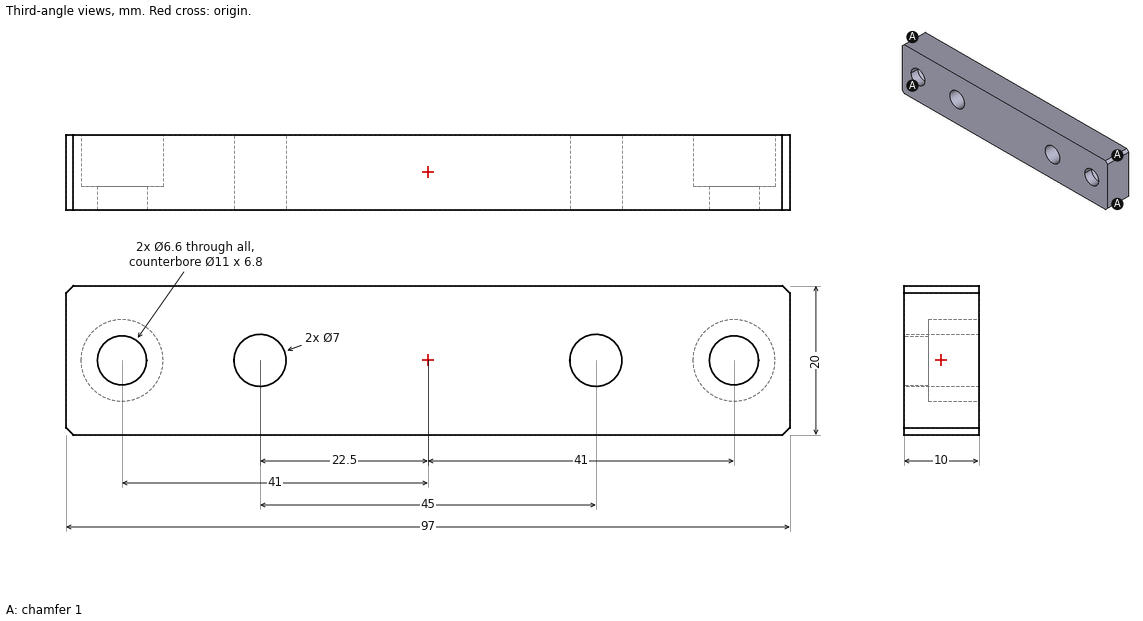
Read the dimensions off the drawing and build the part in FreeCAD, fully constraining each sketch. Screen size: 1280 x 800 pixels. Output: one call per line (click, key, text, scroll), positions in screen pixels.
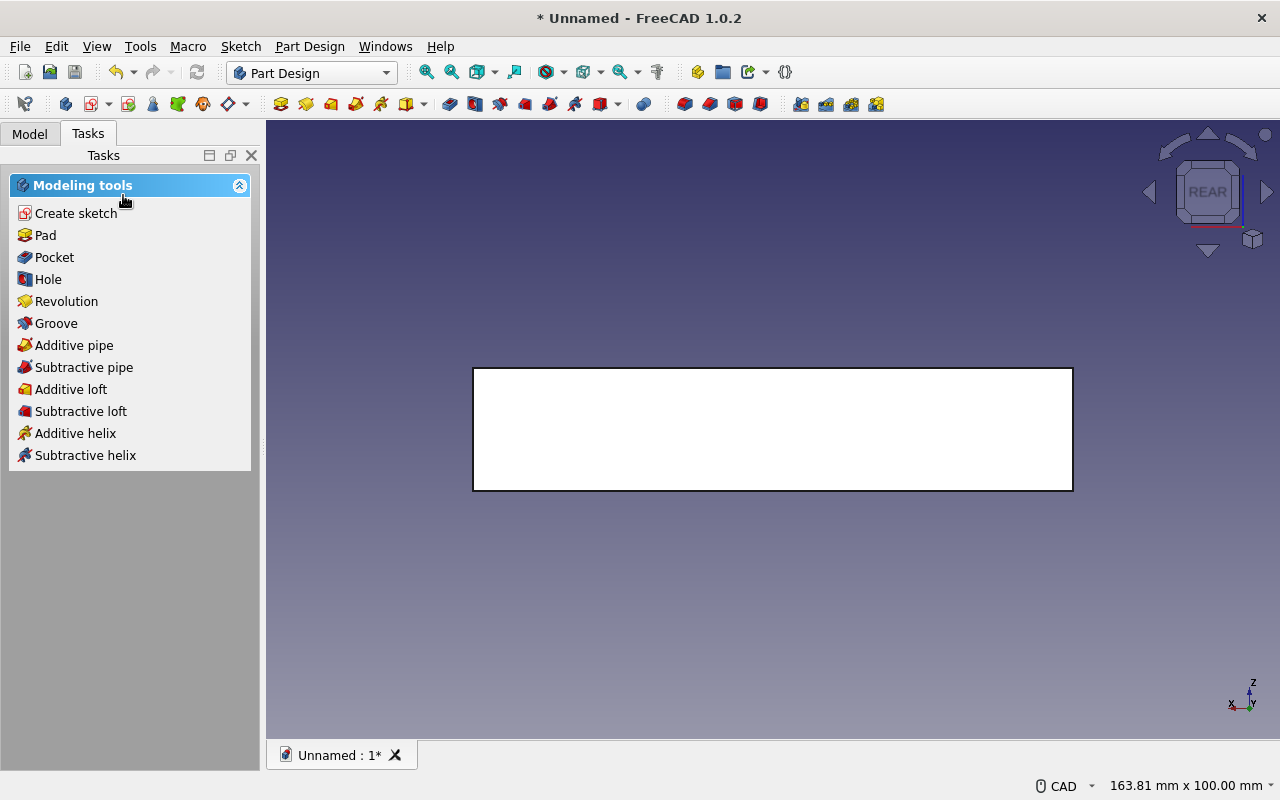
click(450, 104)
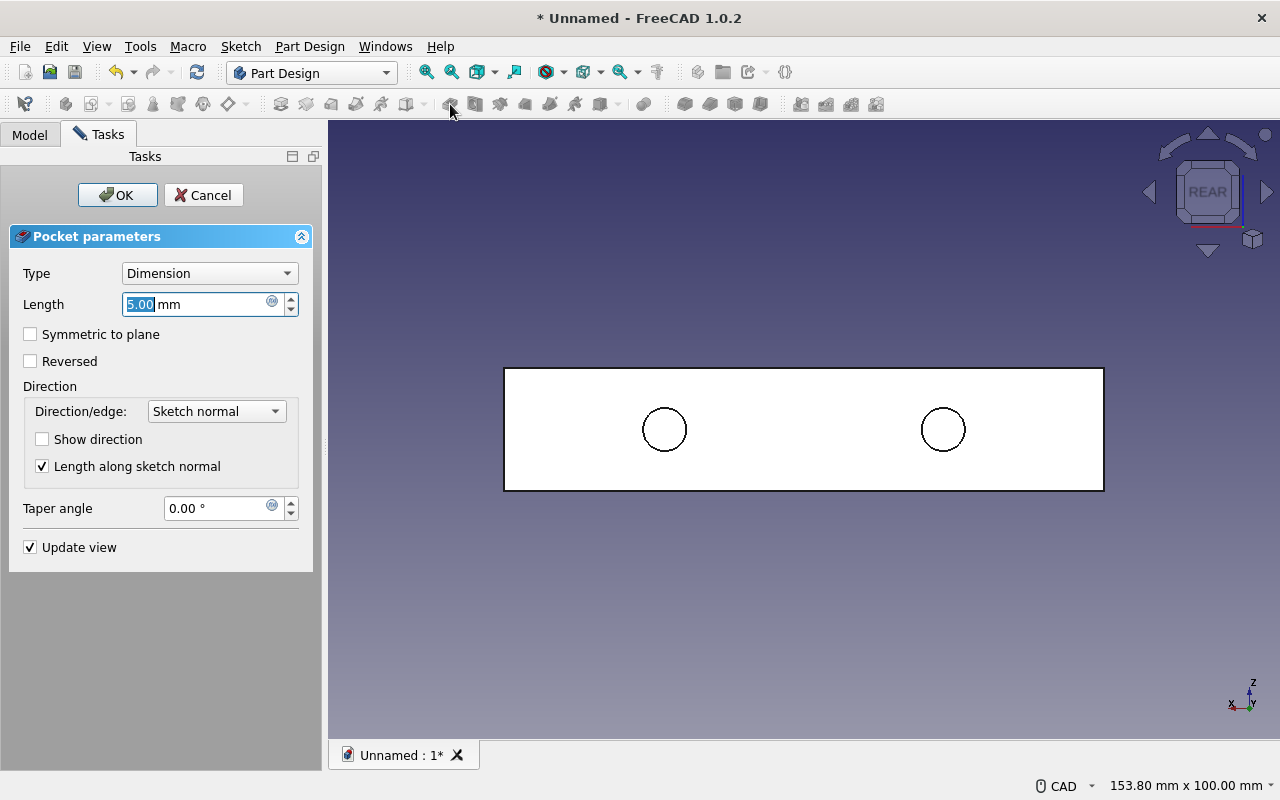
click(210, 274)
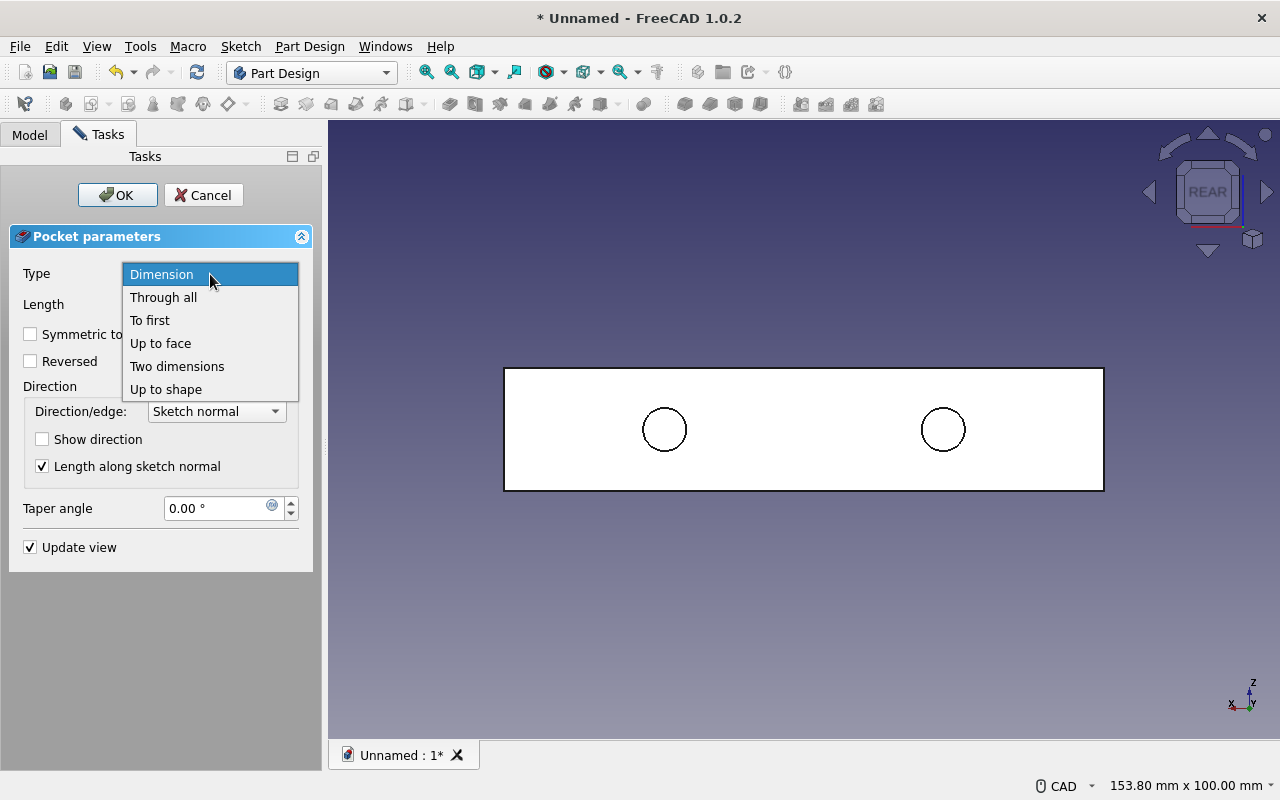
click(208, 298)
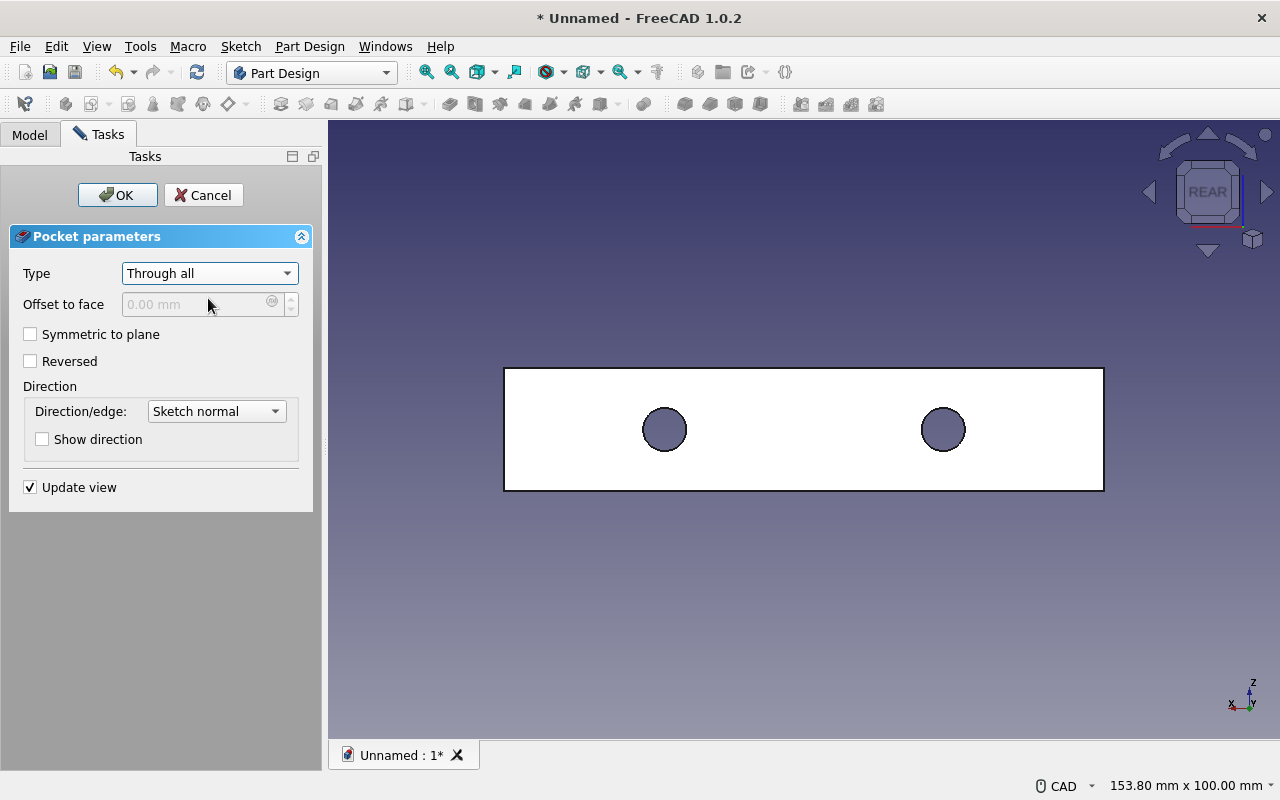
click(118, 195)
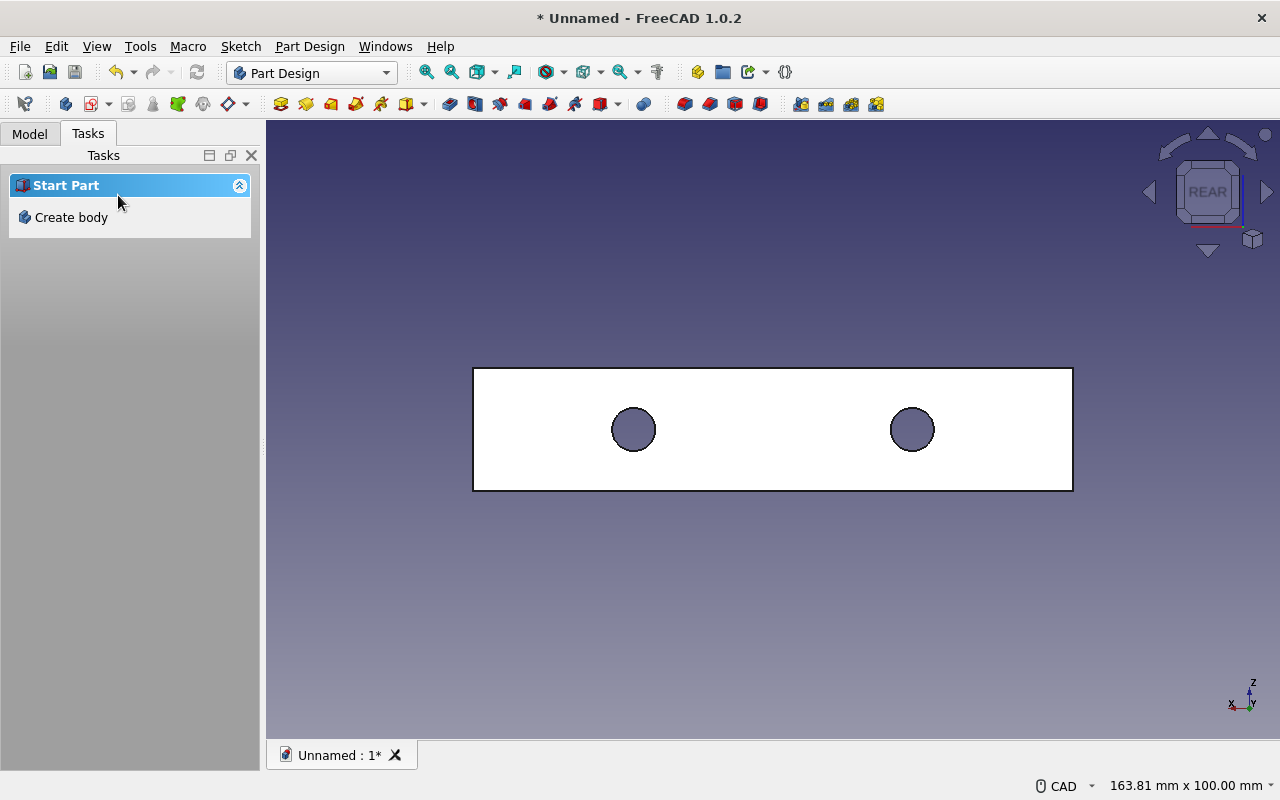
click(773, 428)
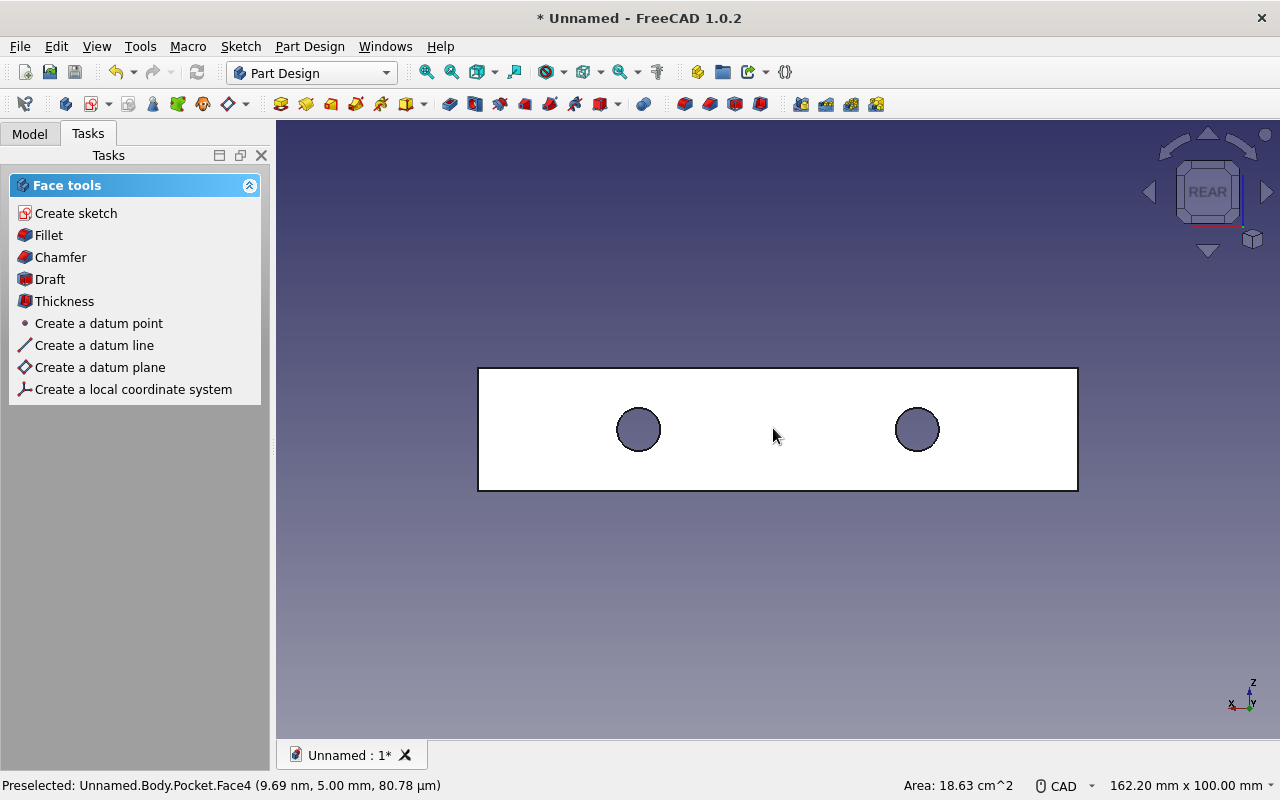
click(90, 104)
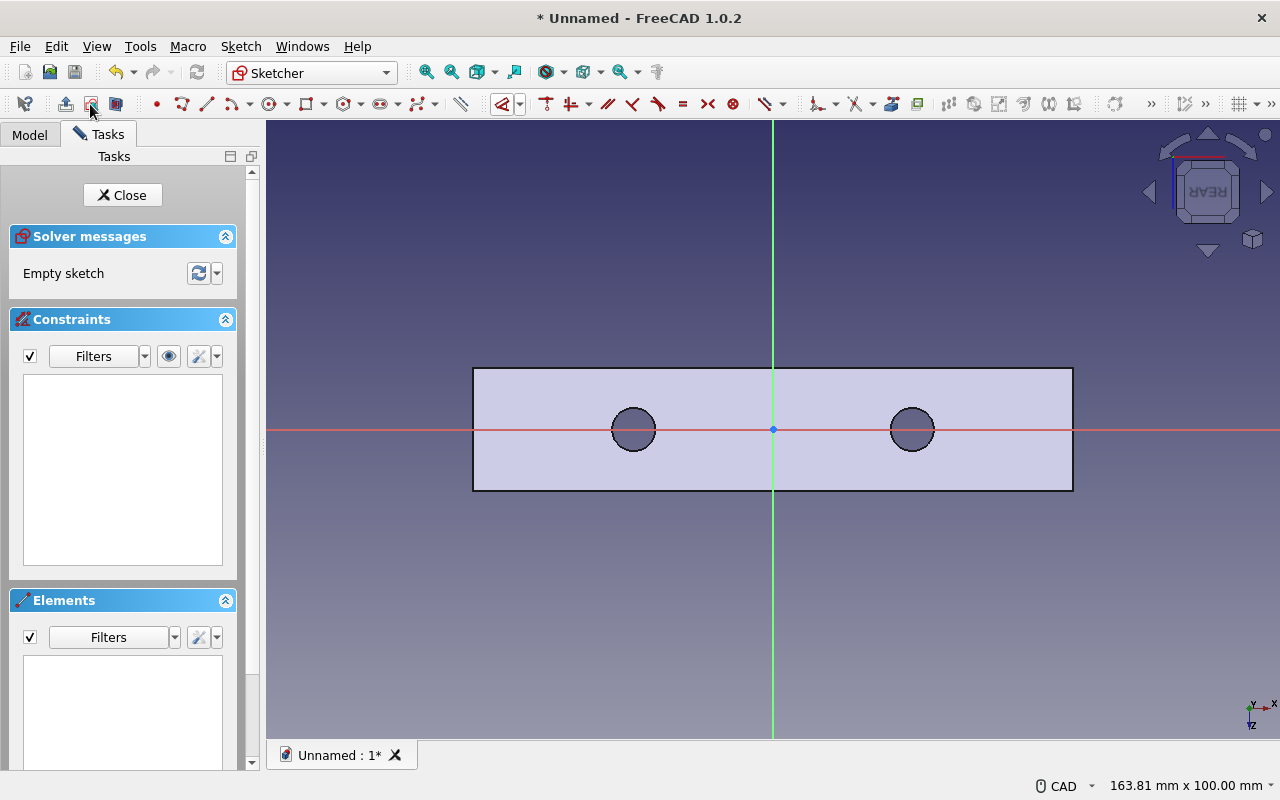
click(268, 104)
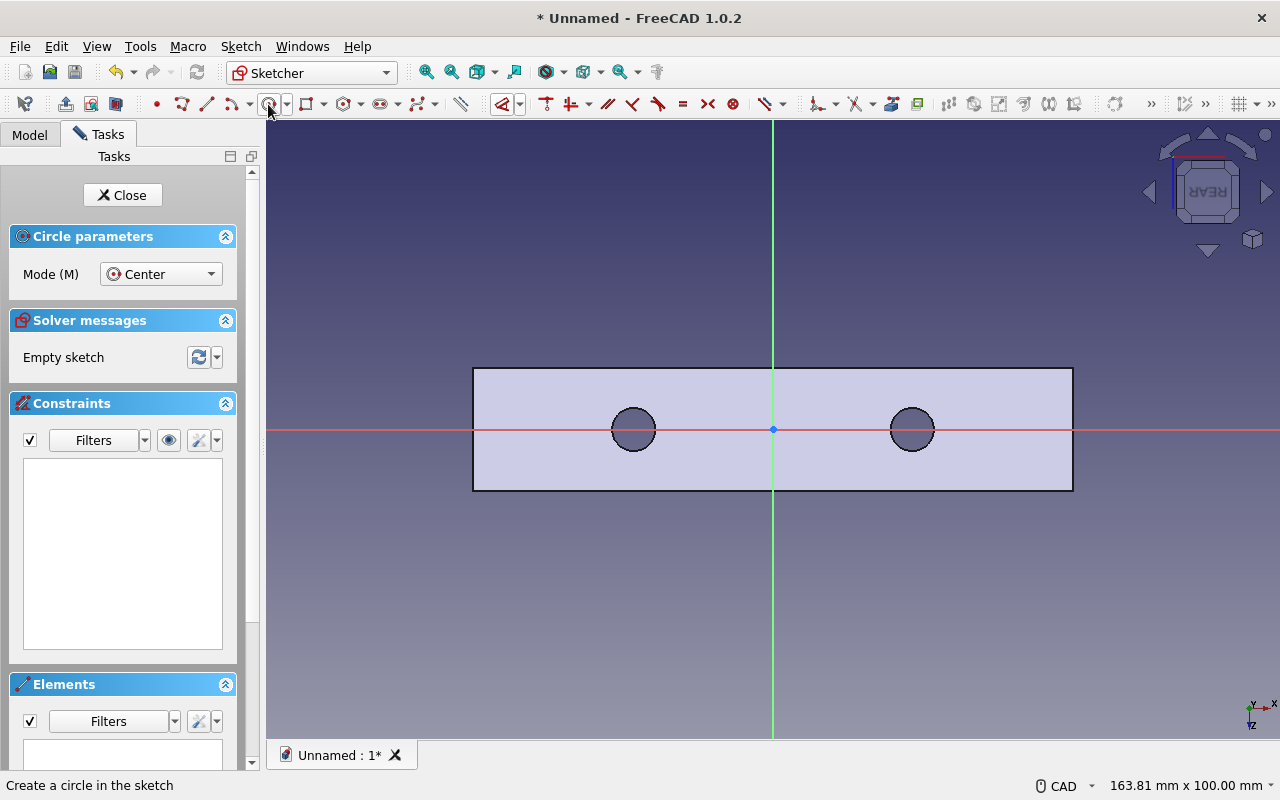
click(519, 429)
click(534, 415)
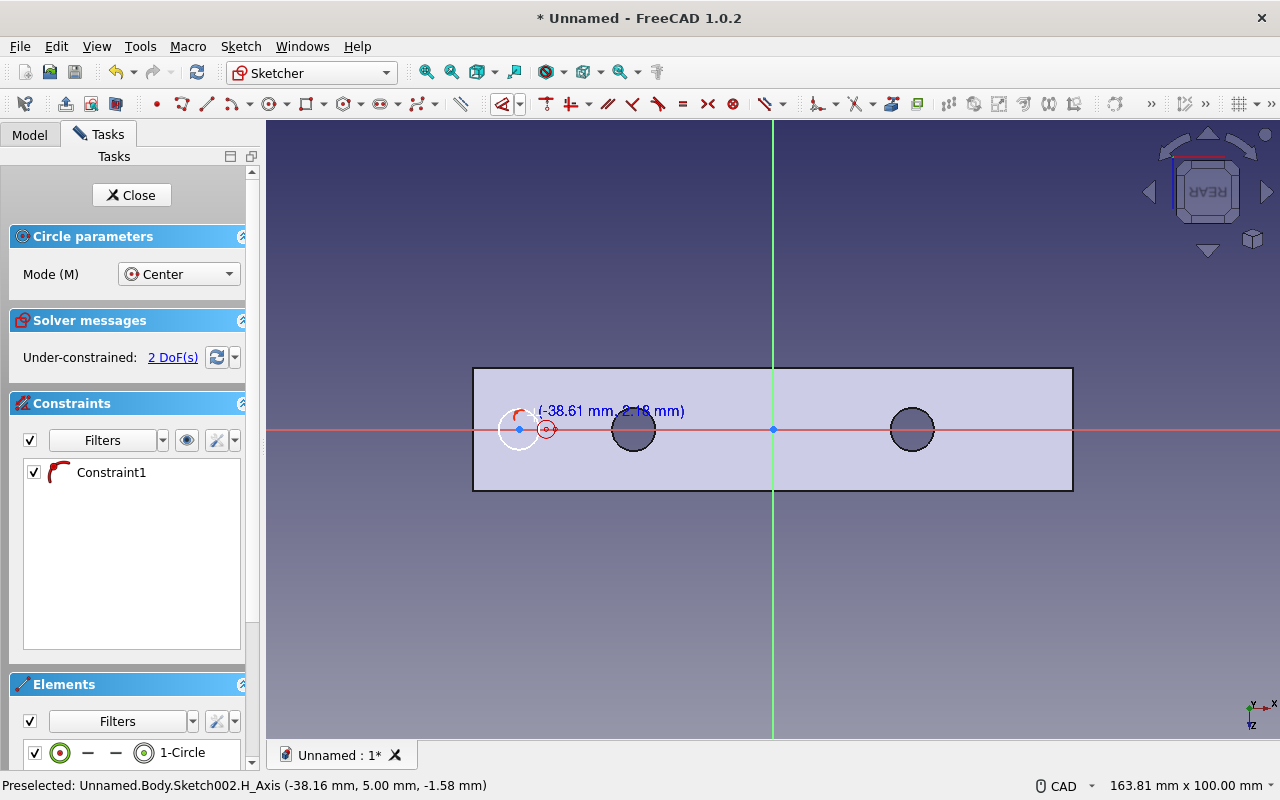
click(1027, 429)
click(1041, 415)
key(Escape)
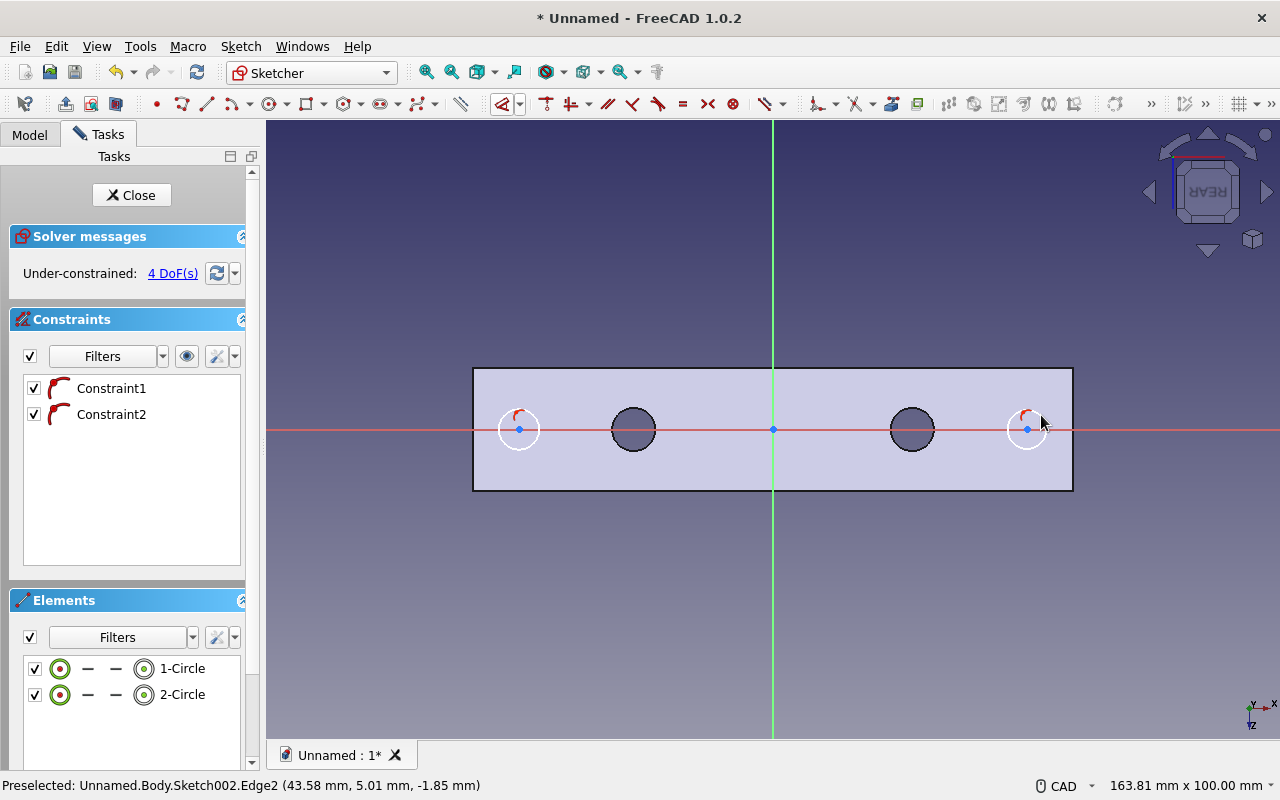
click(533, 415)